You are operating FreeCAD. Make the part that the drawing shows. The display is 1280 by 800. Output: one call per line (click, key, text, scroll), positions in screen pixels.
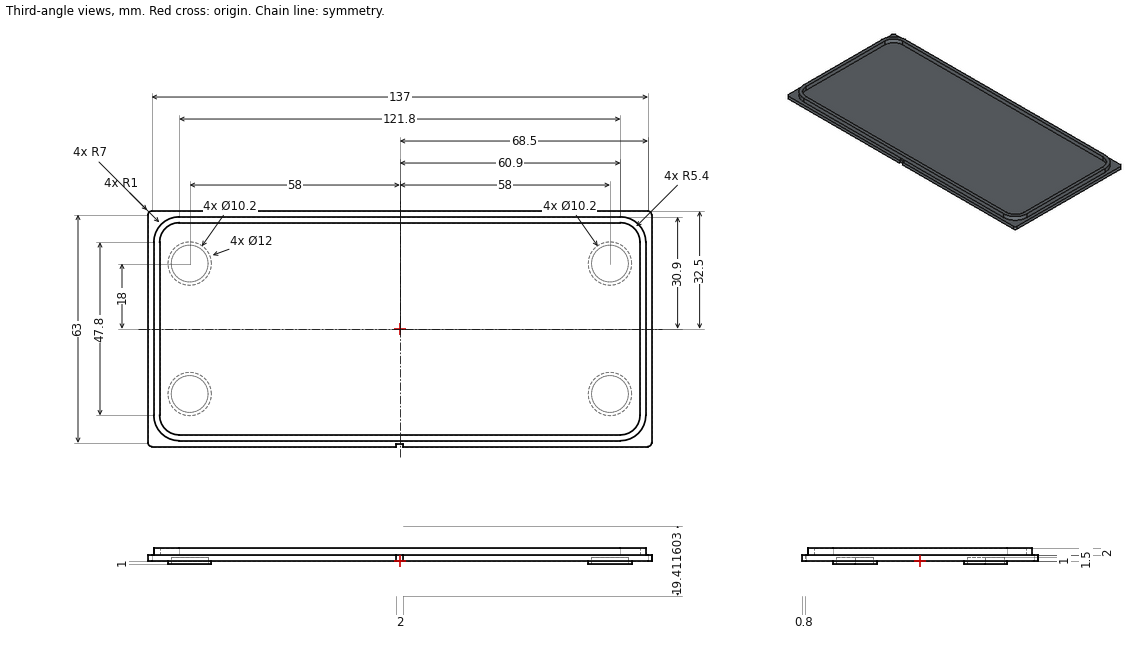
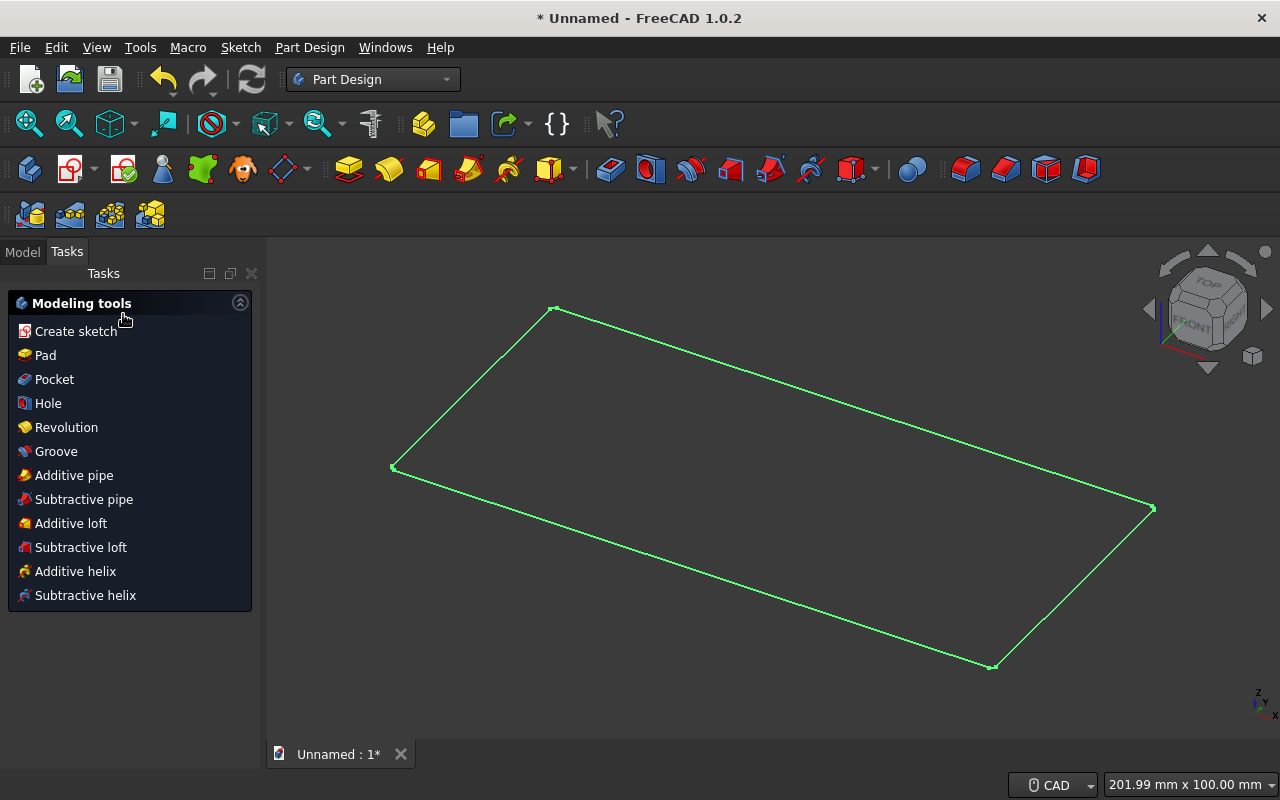
click(350, 170)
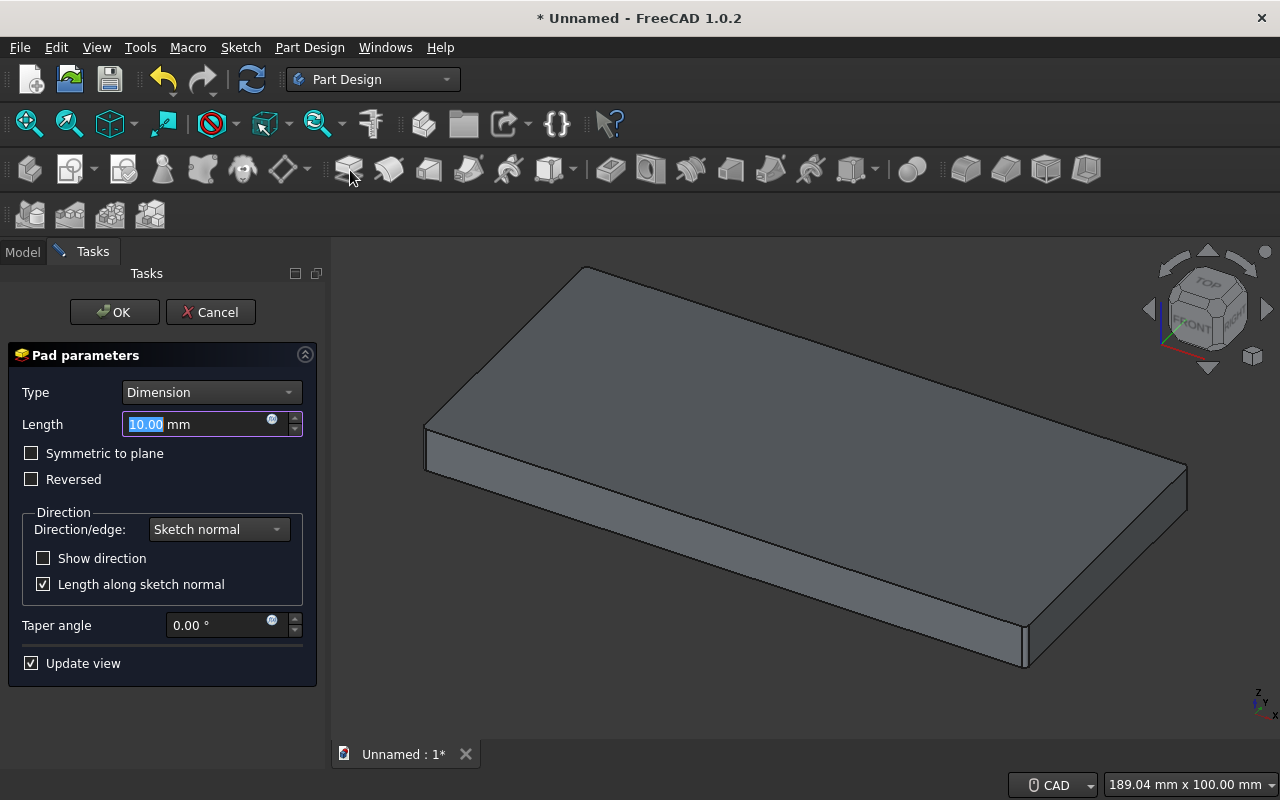
text(1.5)
key(Tab)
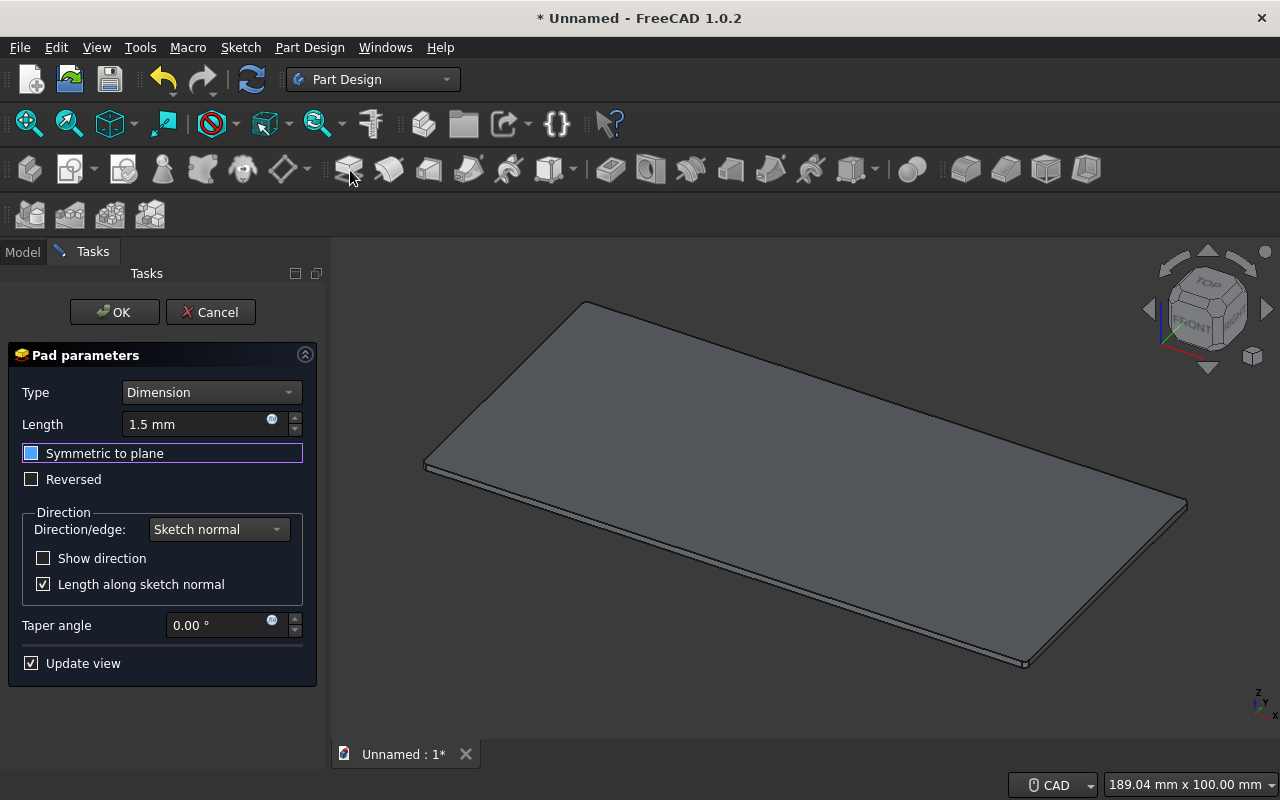
click(115, 312)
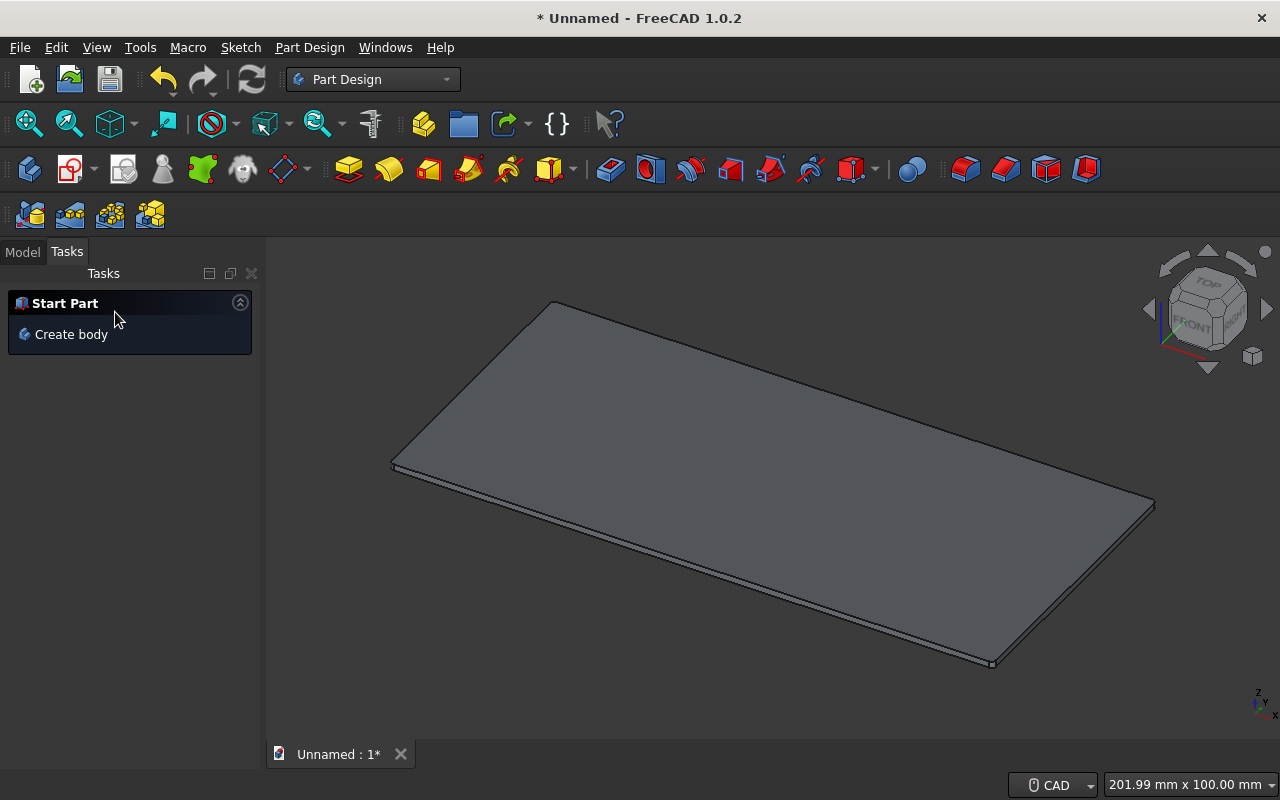
key(5)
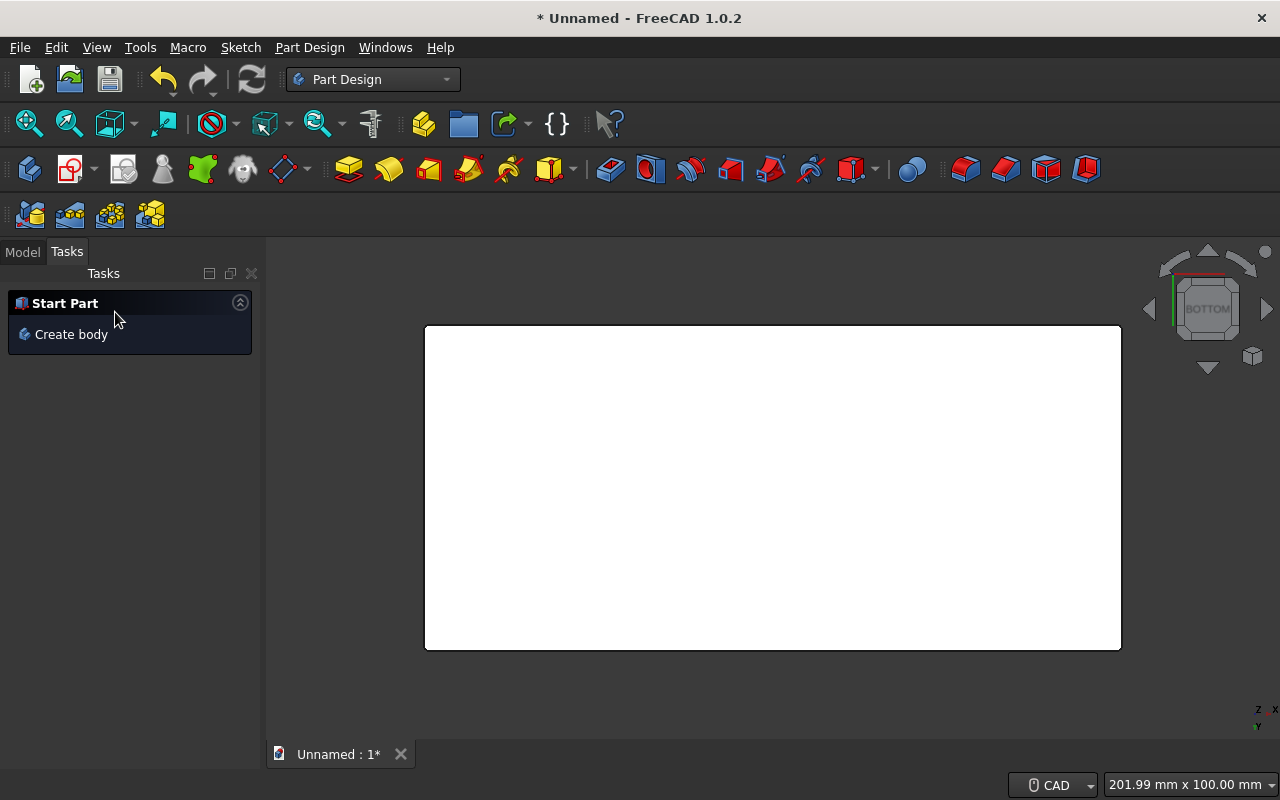
click(873, 487)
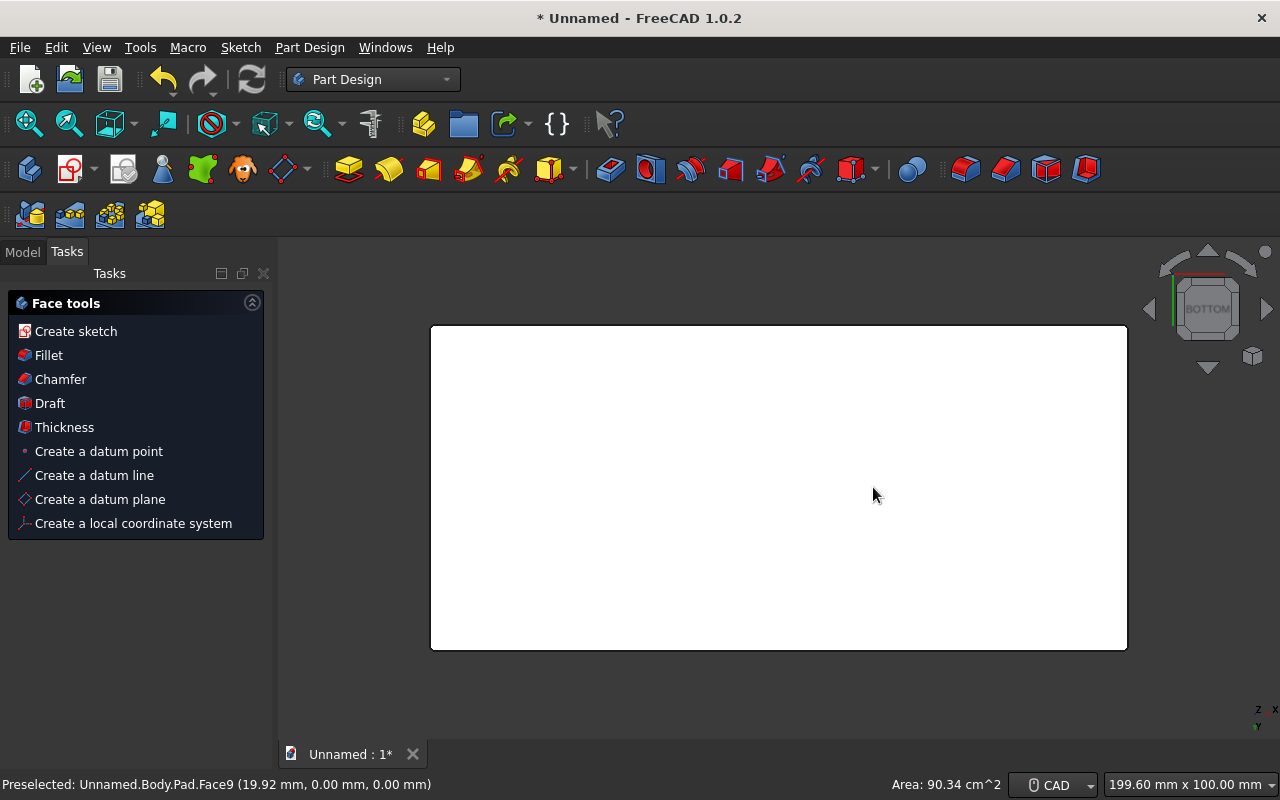
click(70, 170)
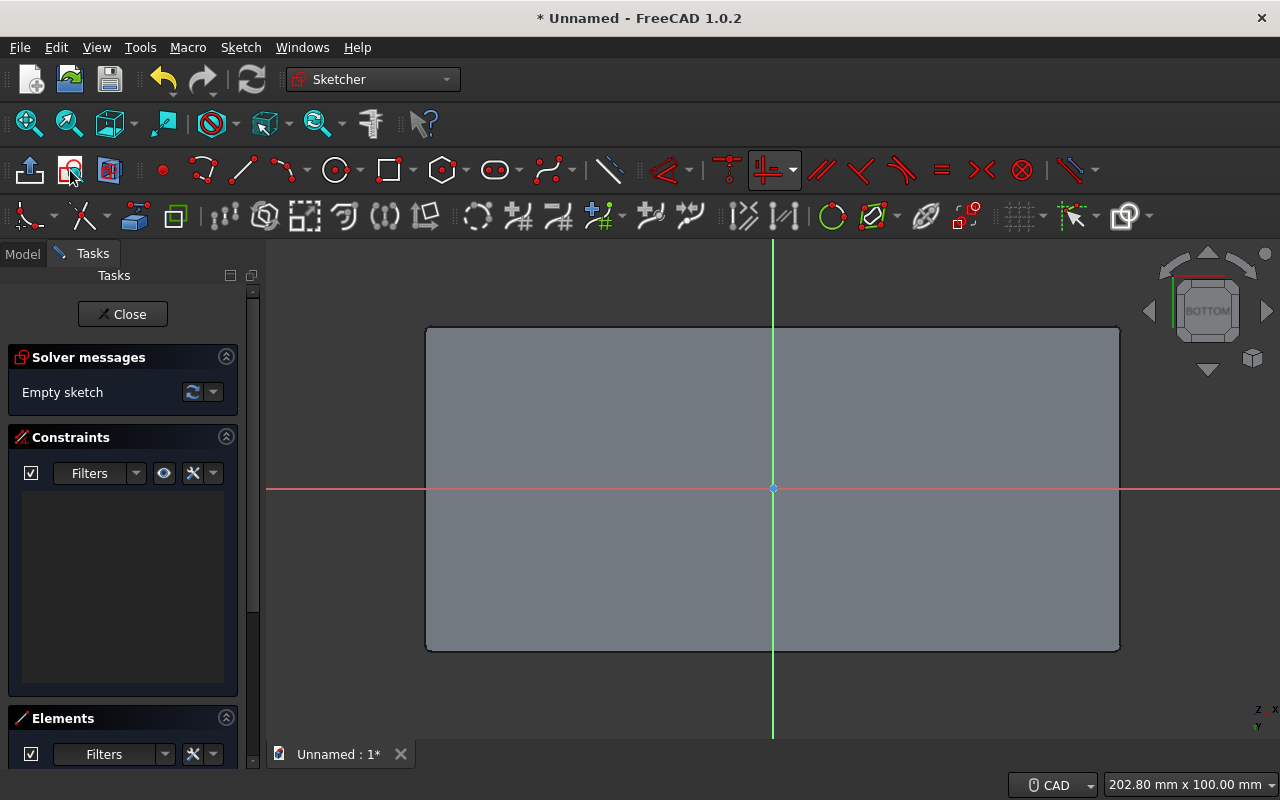
scroll(395, 489, down, 1)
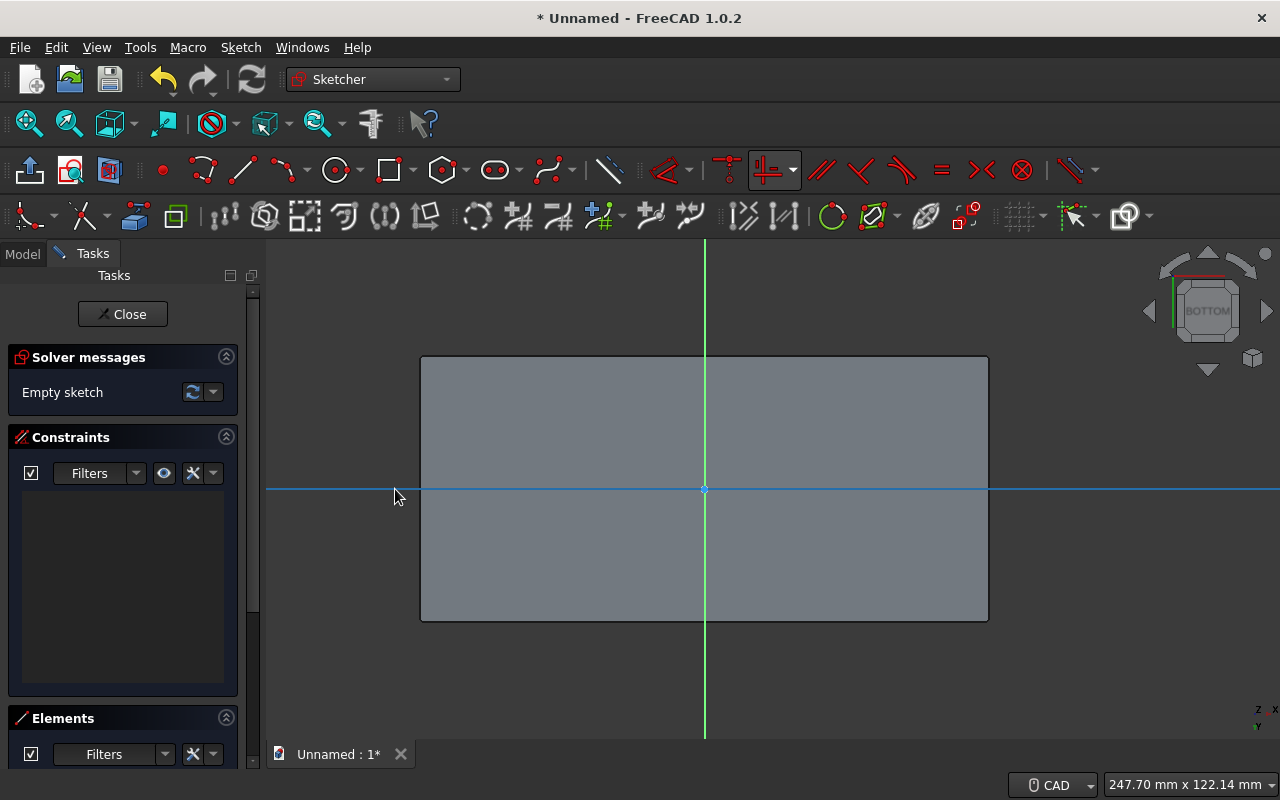
click(336, 170)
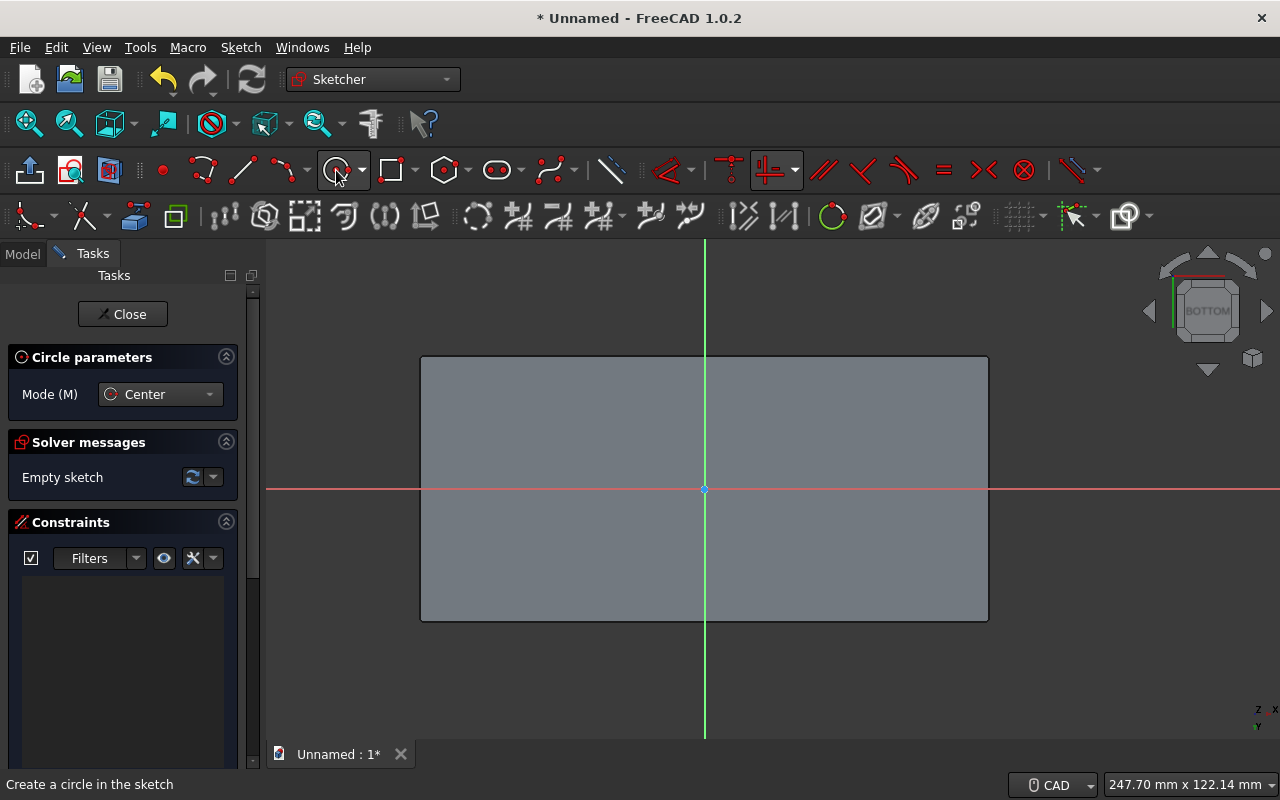
click(467, 563)
move(484, 545)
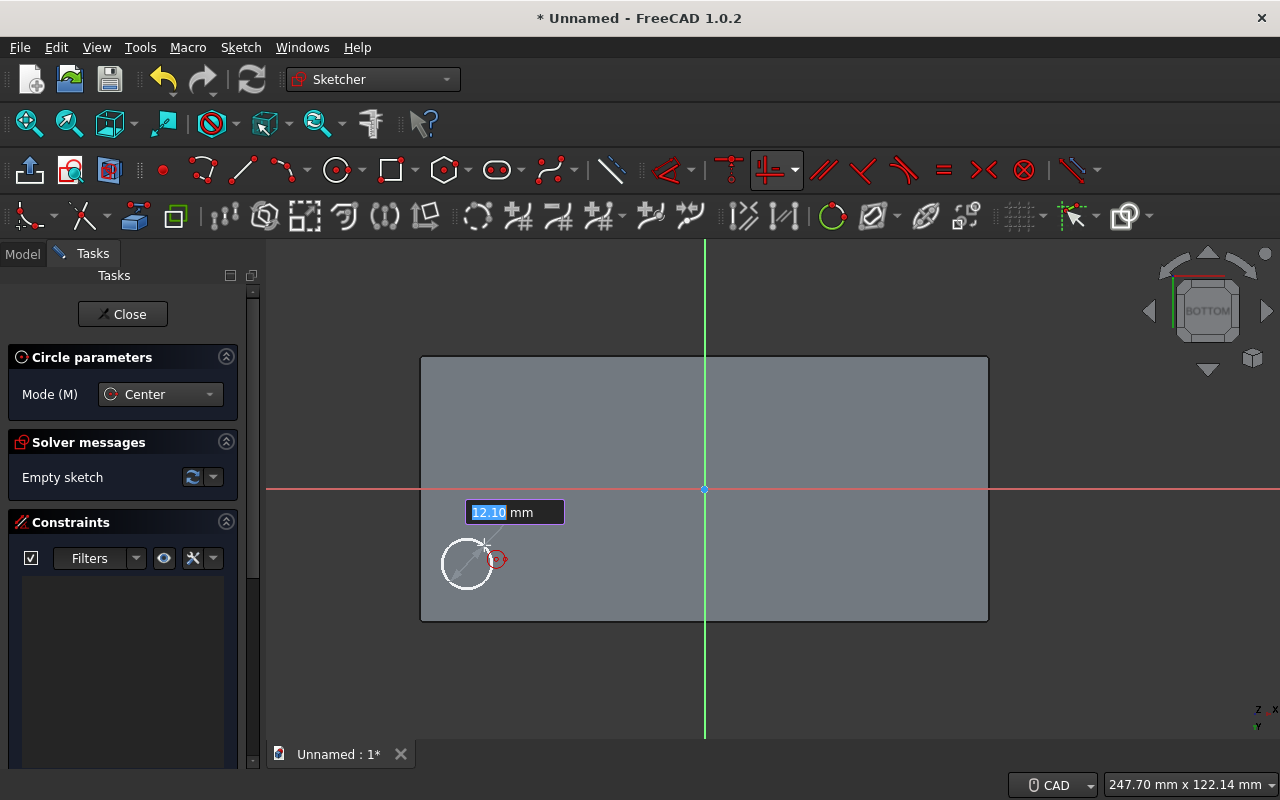
text(12)
key(Return)